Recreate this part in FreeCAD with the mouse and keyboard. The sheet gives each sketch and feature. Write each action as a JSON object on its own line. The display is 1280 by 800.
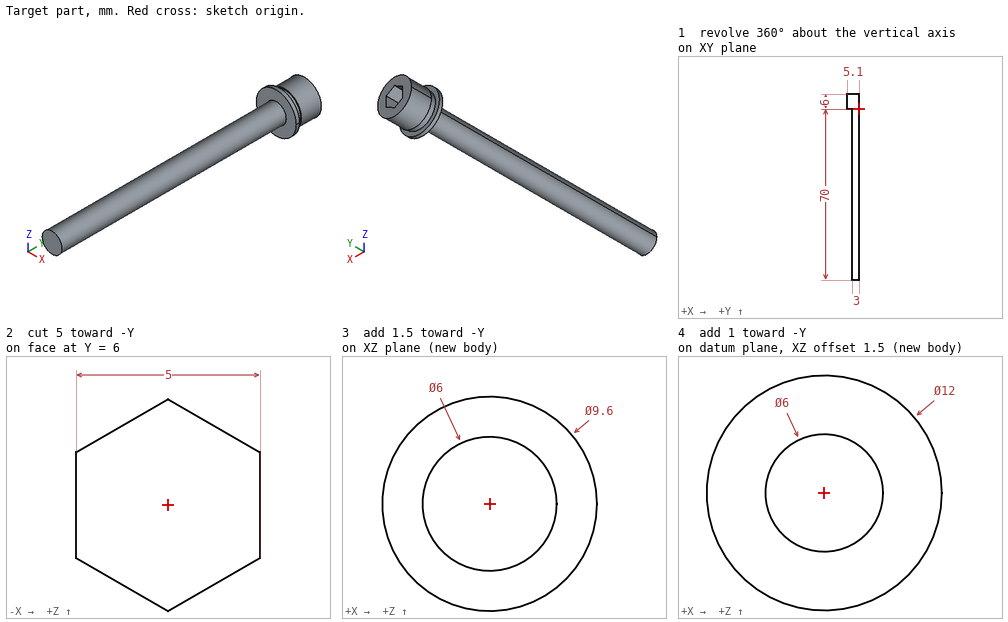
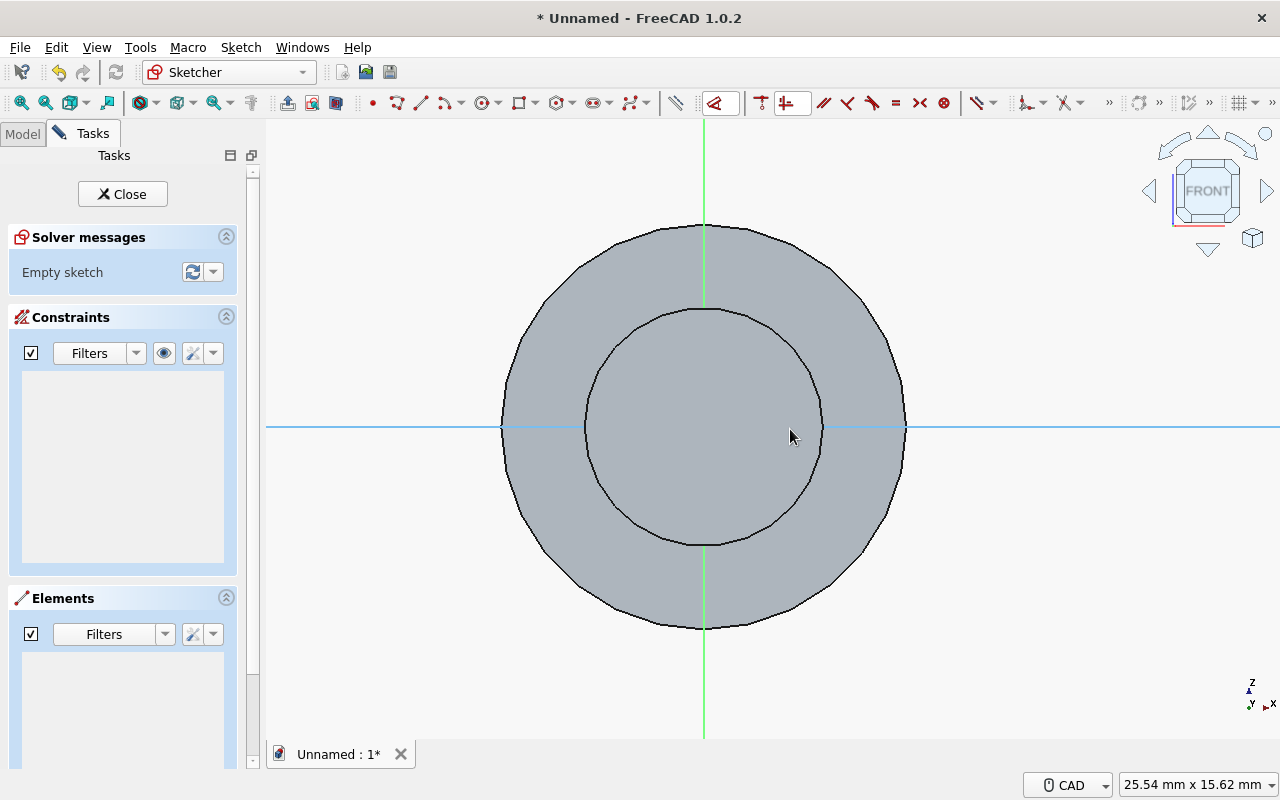
{"action": "left_click", "coordinate": [482, 104]}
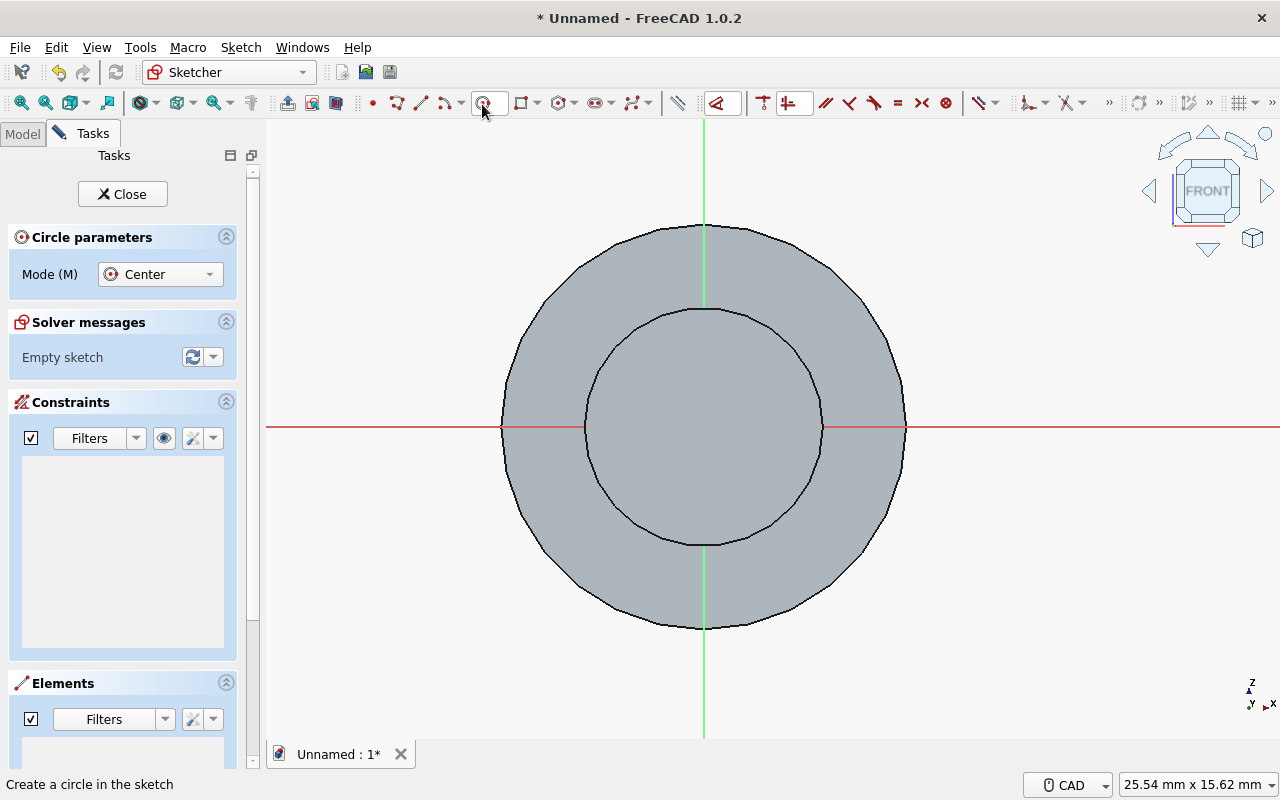
{"action": "left_click", "coordinate": [704, 427]}
{"action": "left_click", "coordinate": [838, 292]}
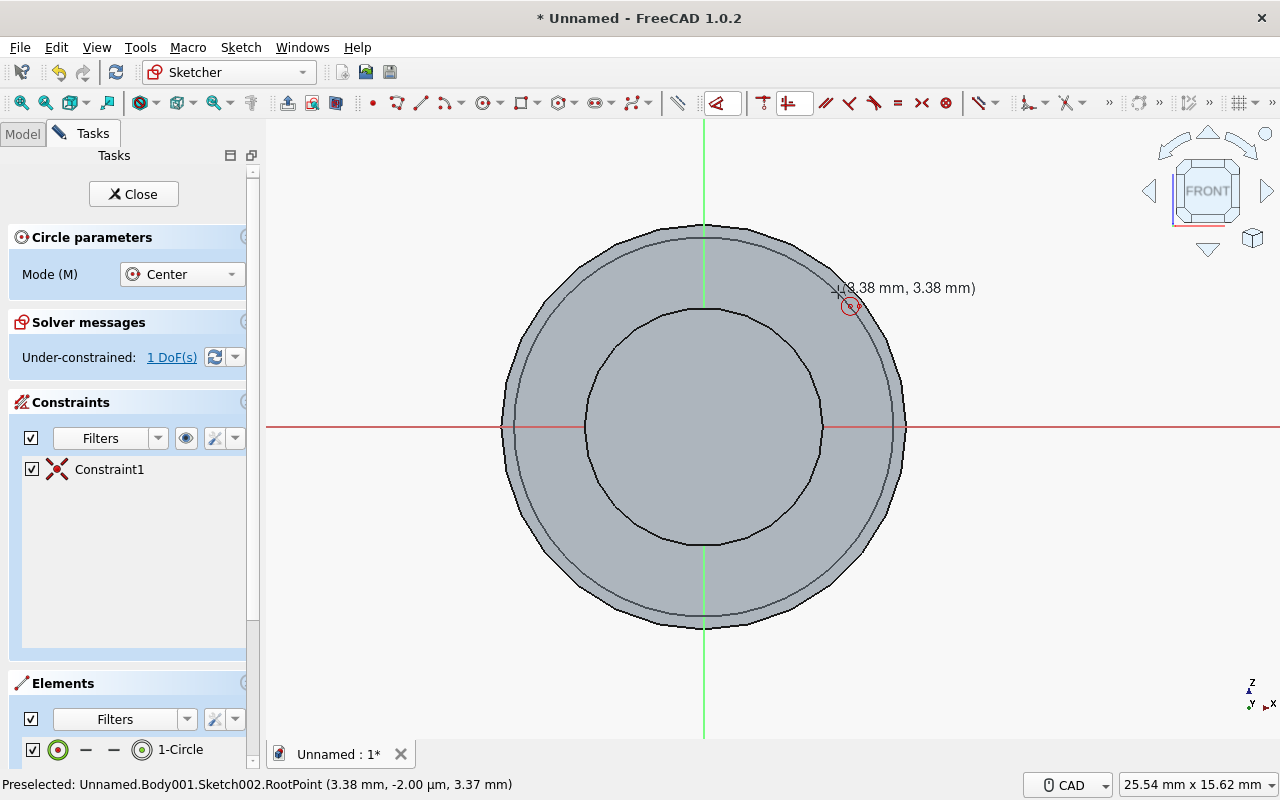
{"action": "left_click", "coordinate": [704, 427]}
{"action": "left_click", "coordinate": [788, 343]}
{"action": "key", "text": "Escape"}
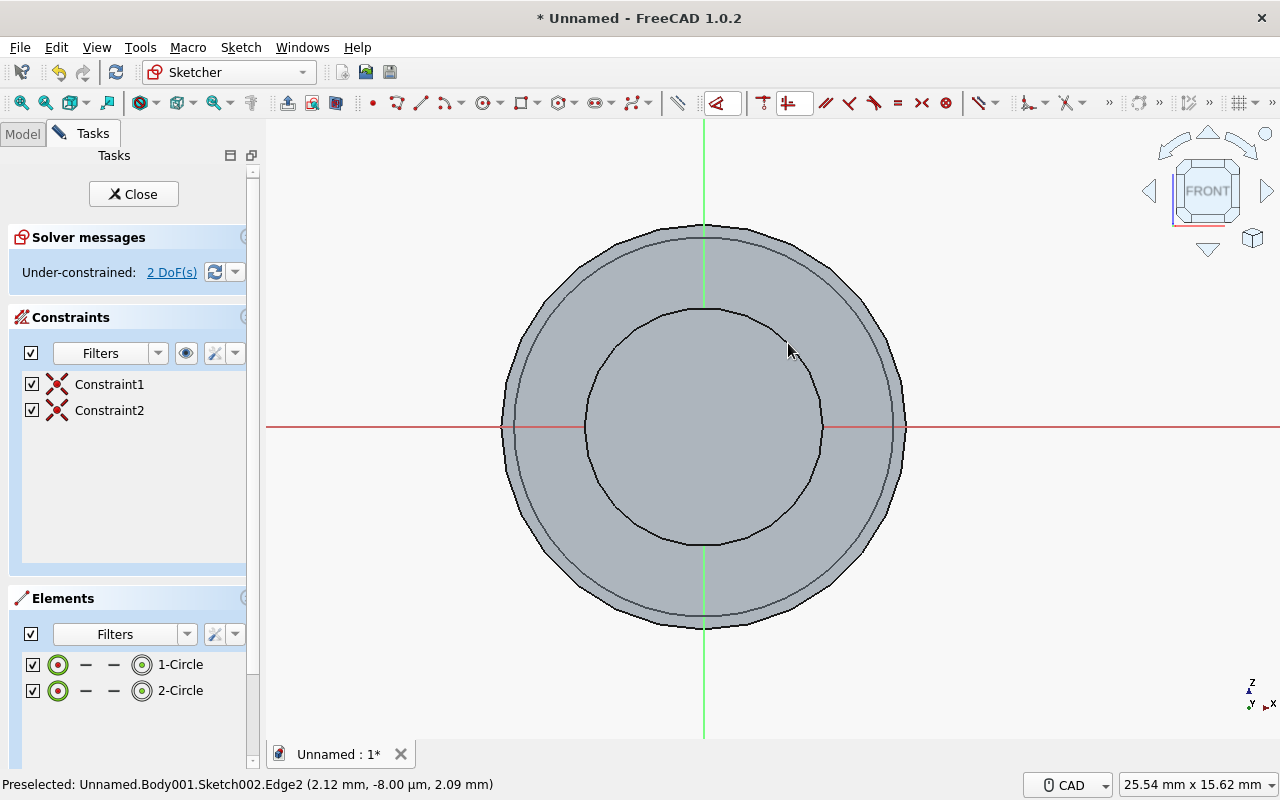
{"action": "left_click", "coordinate": [837, 292]}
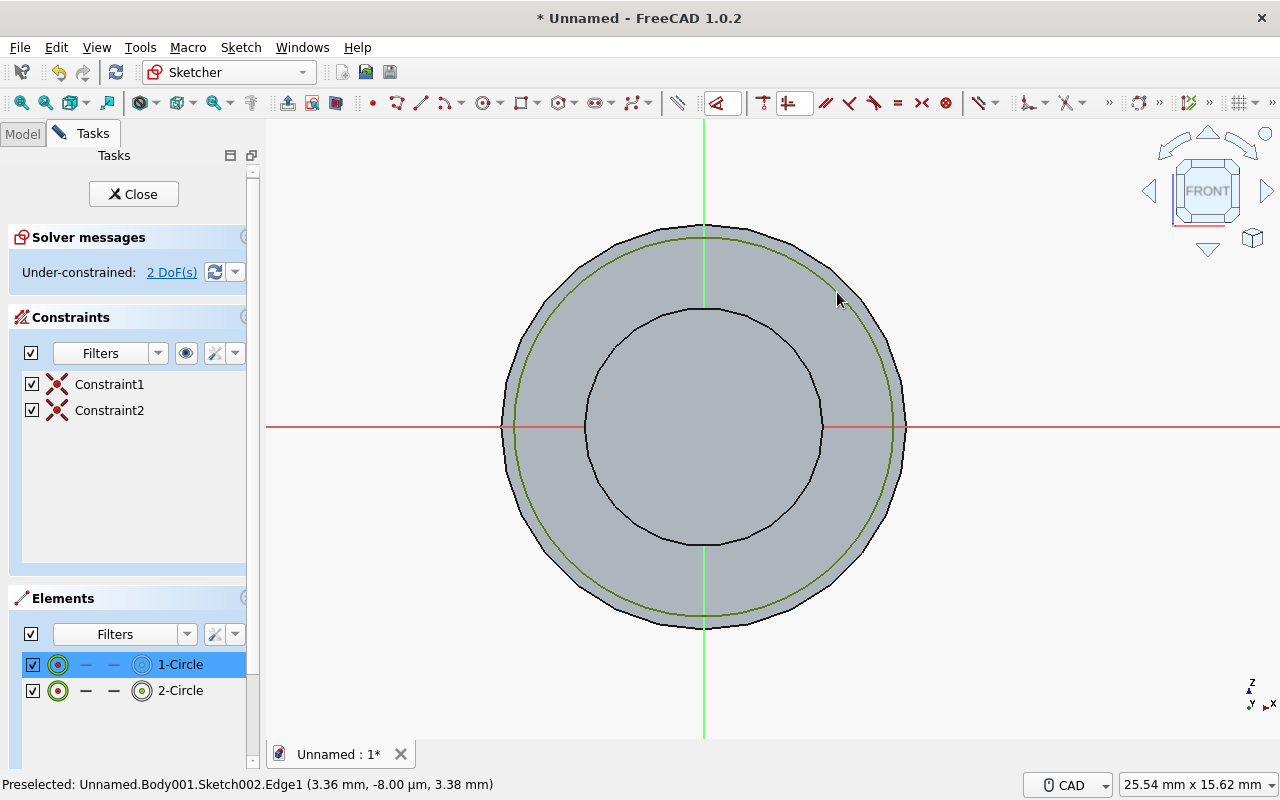
{"action": "key", "text": "k o"}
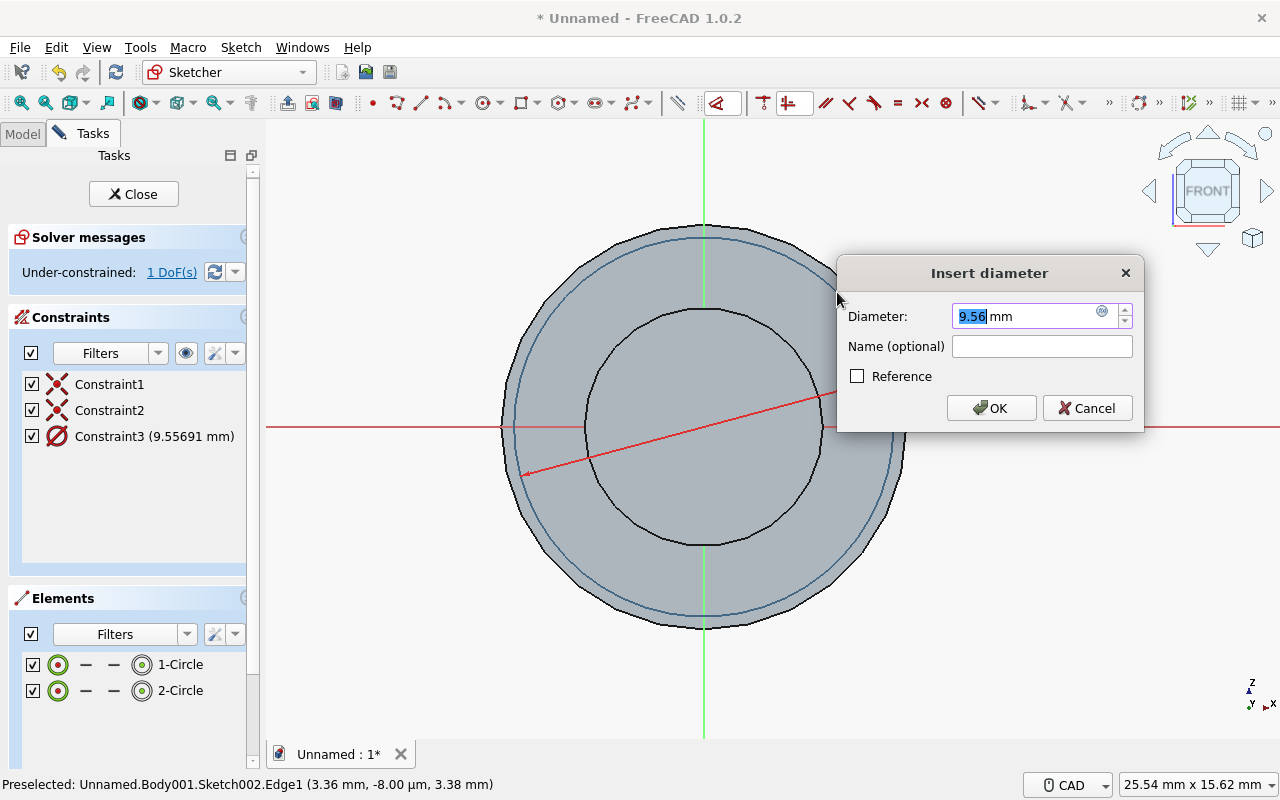
{"action": "type", "text": "9.6"}
{"action": "key", "text": "Return"}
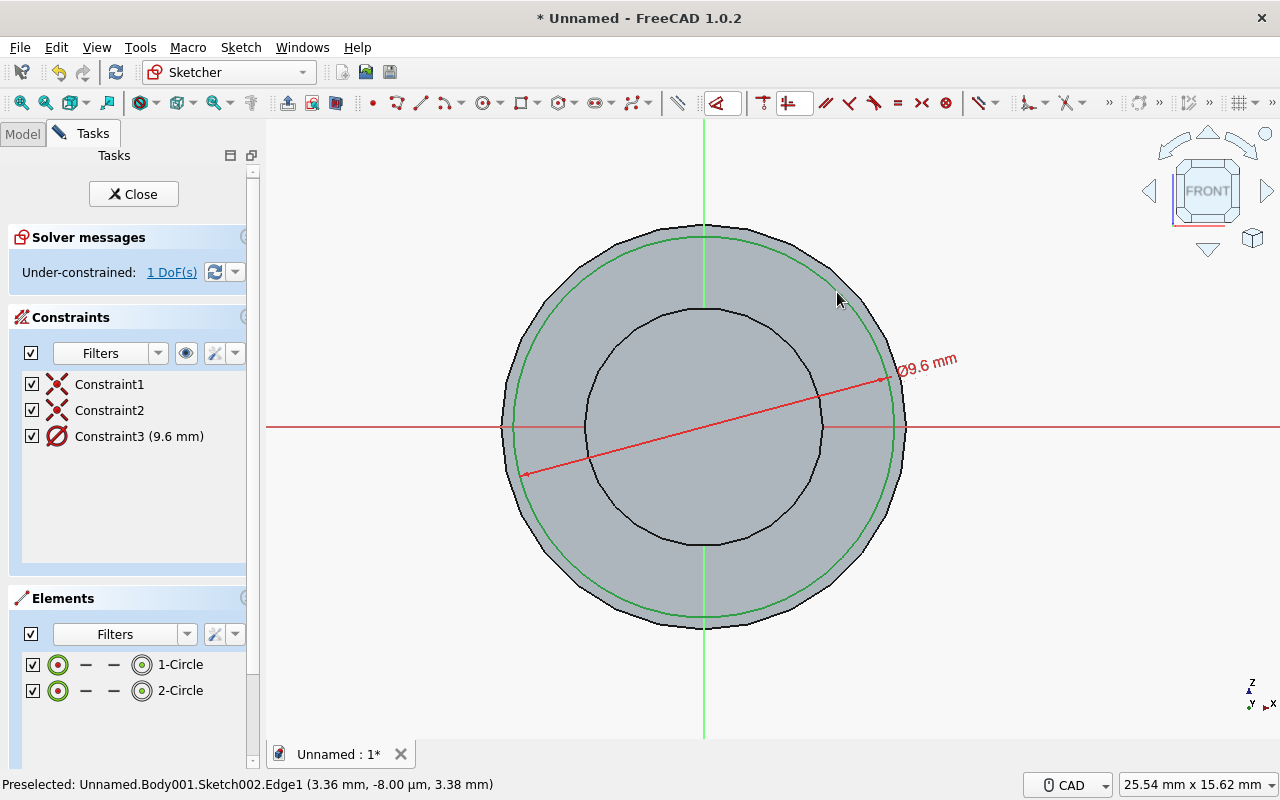
{"action": "left_click", "coordinate": [787, 343]}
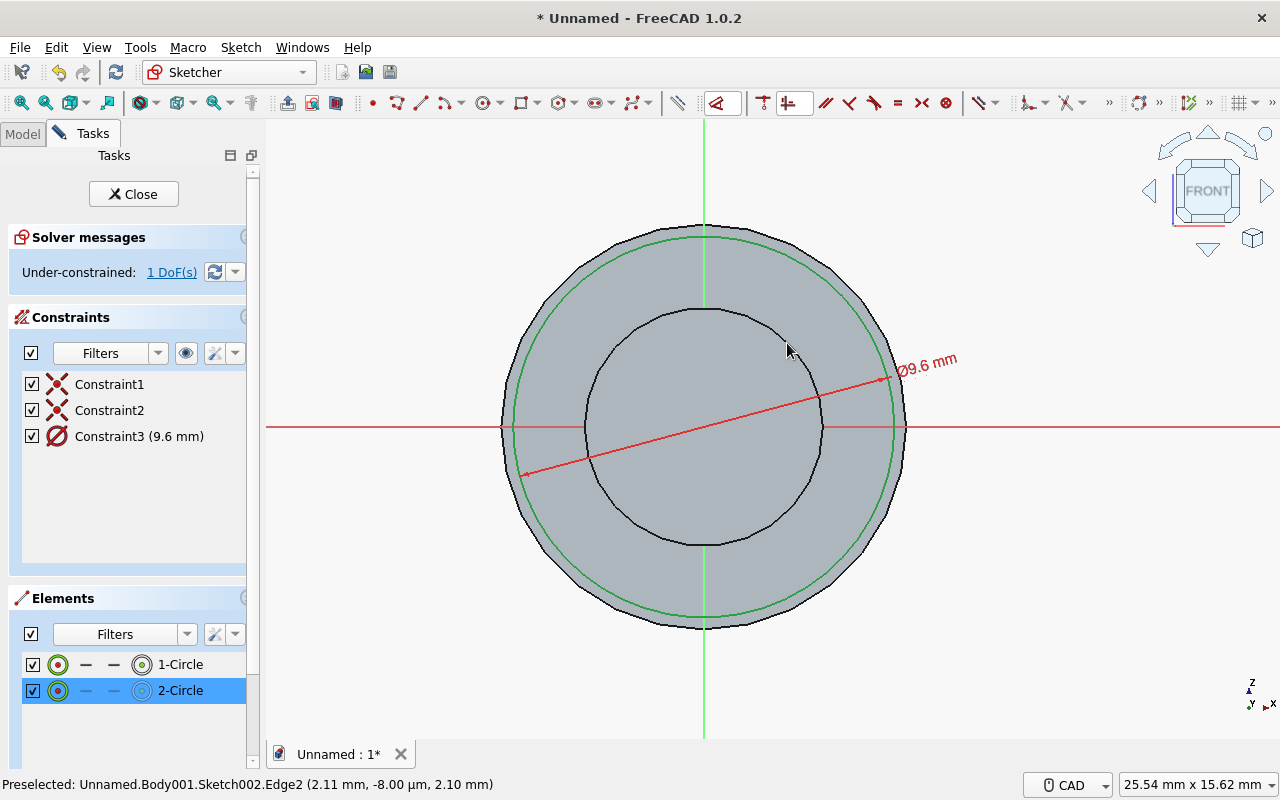
{"action": "key", "text": "k o"}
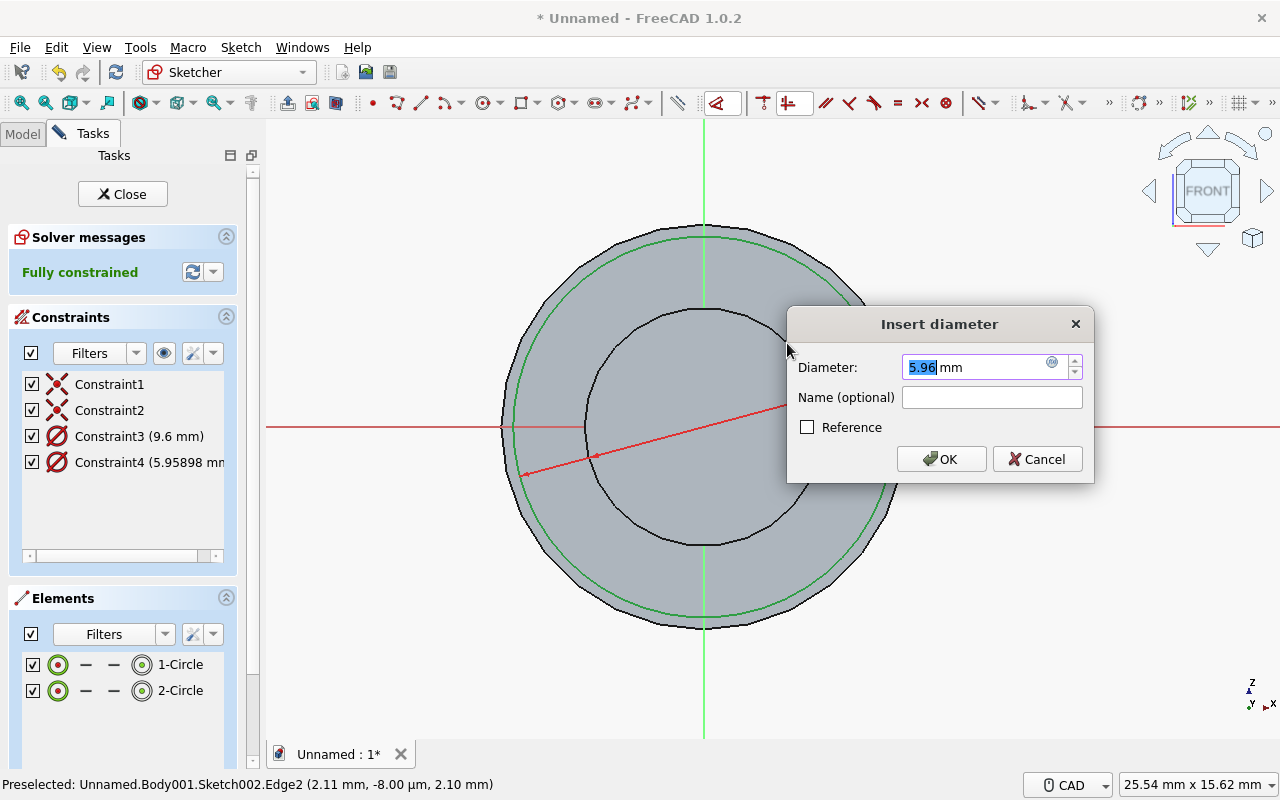
{"action": "type", "text": "6"}
{"action": "key", "text": "Return"}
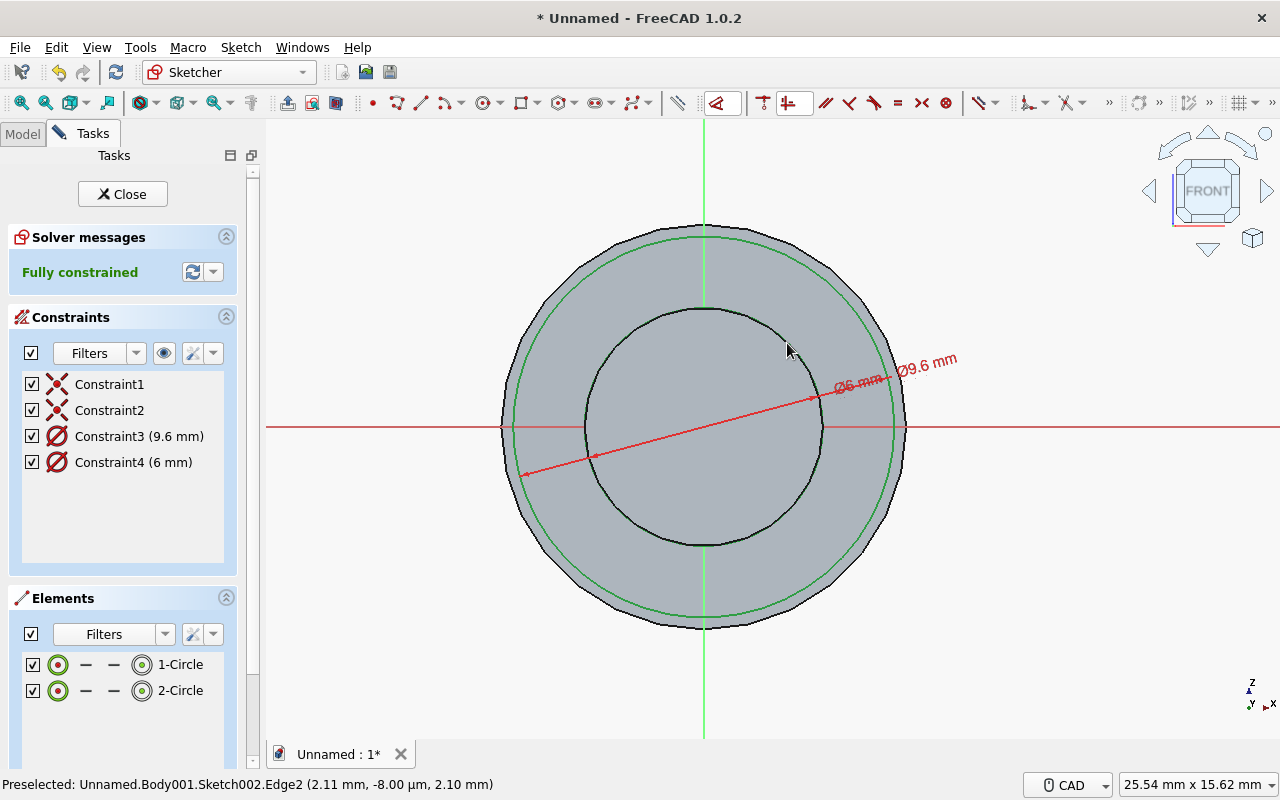
{"action": "left_click", "coordinate": [123, 194]}